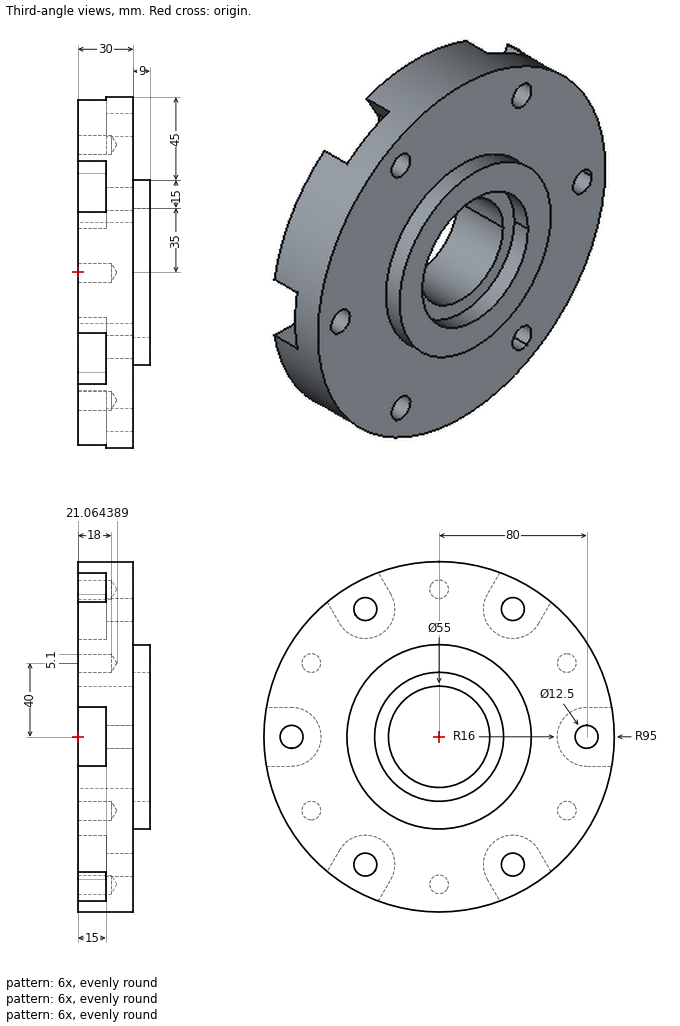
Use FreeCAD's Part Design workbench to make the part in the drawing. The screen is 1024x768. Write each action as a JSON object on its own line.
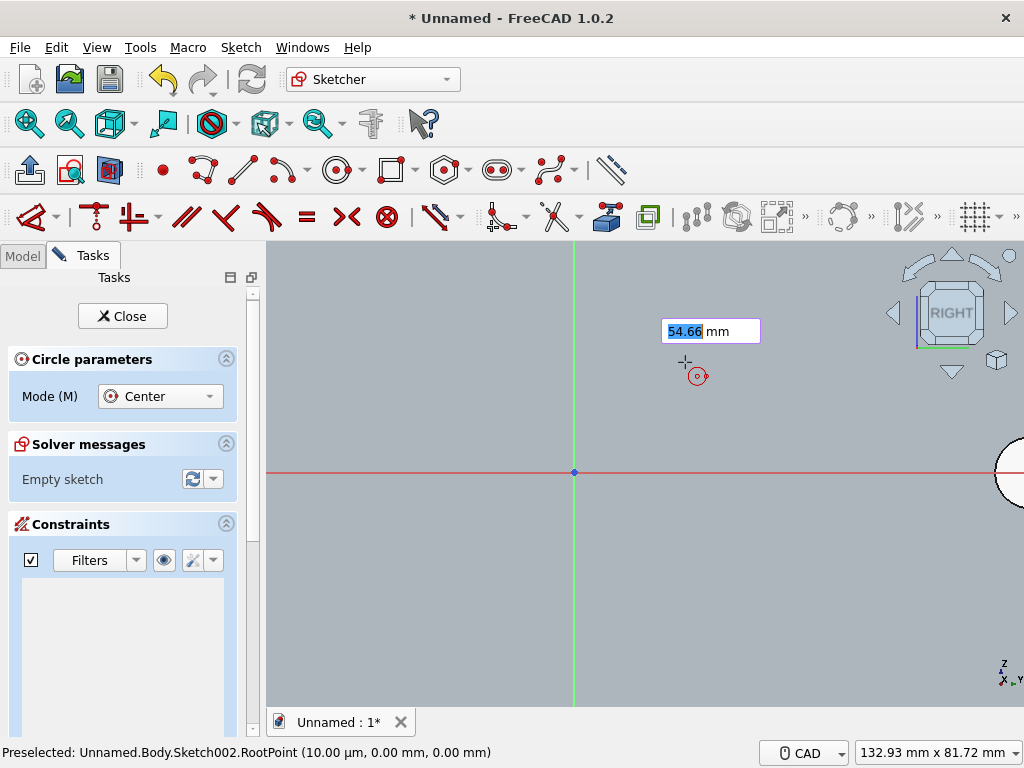
{"action": "type", "text": "55"}
{"action": "key", "text": "Return"}
{"action": "key", "text": "Escape"}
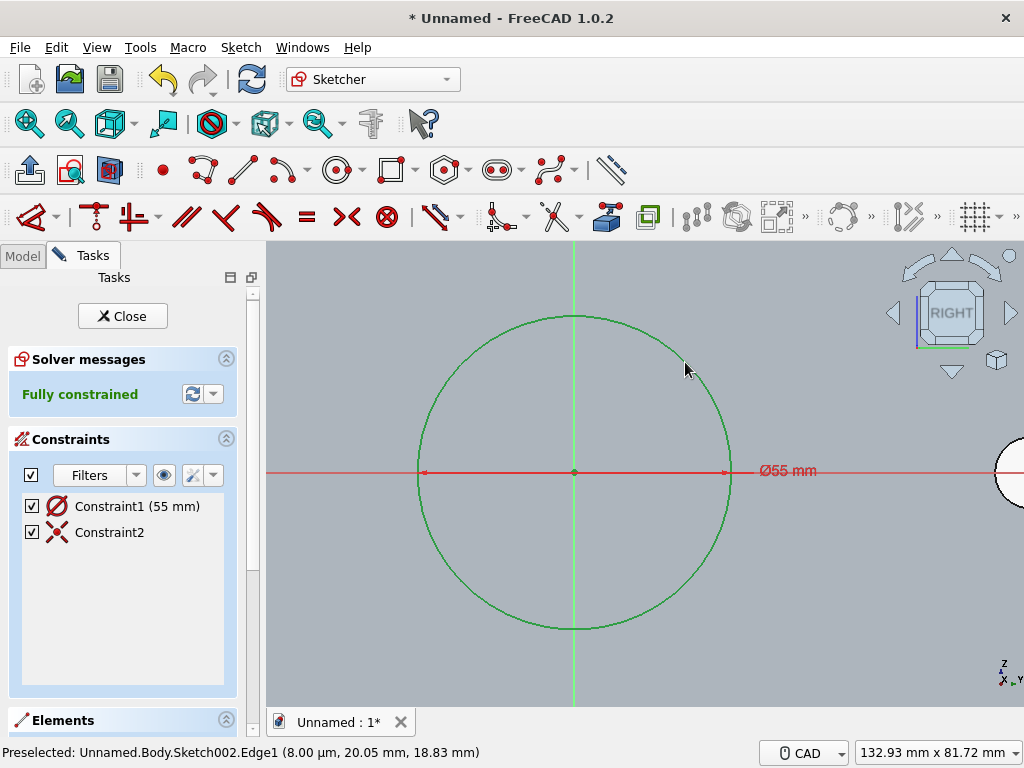
{"action": "left_click", "coordinate": [123, 316]}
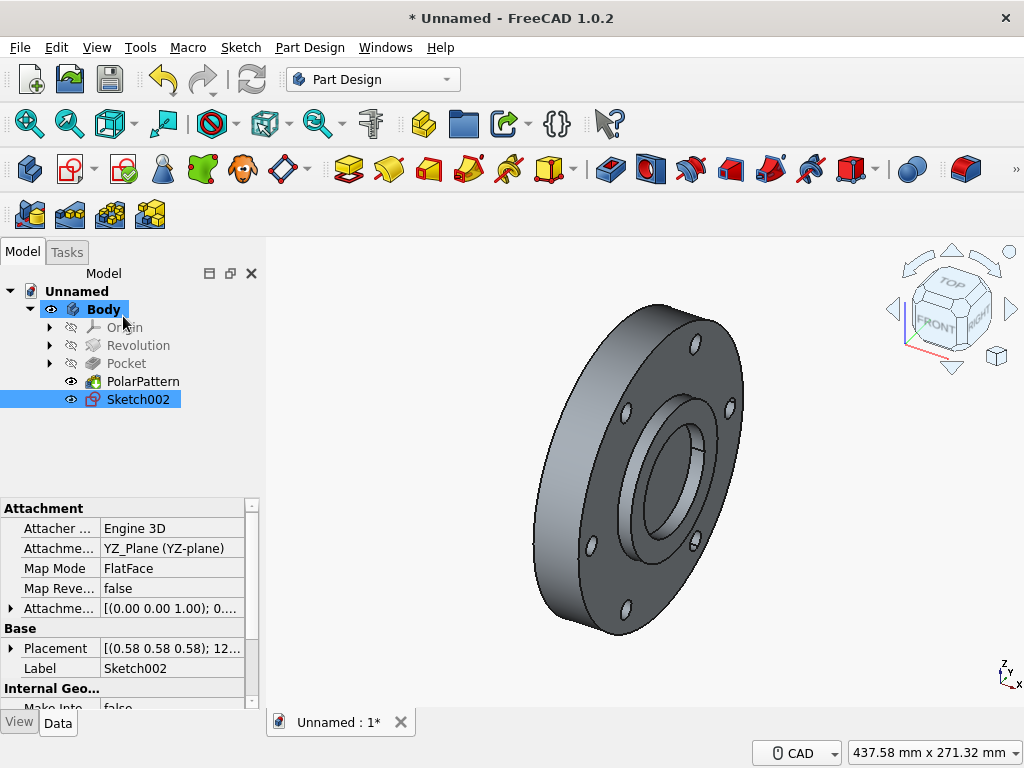
{"action": "left_click", "coordinate": [612, 170]}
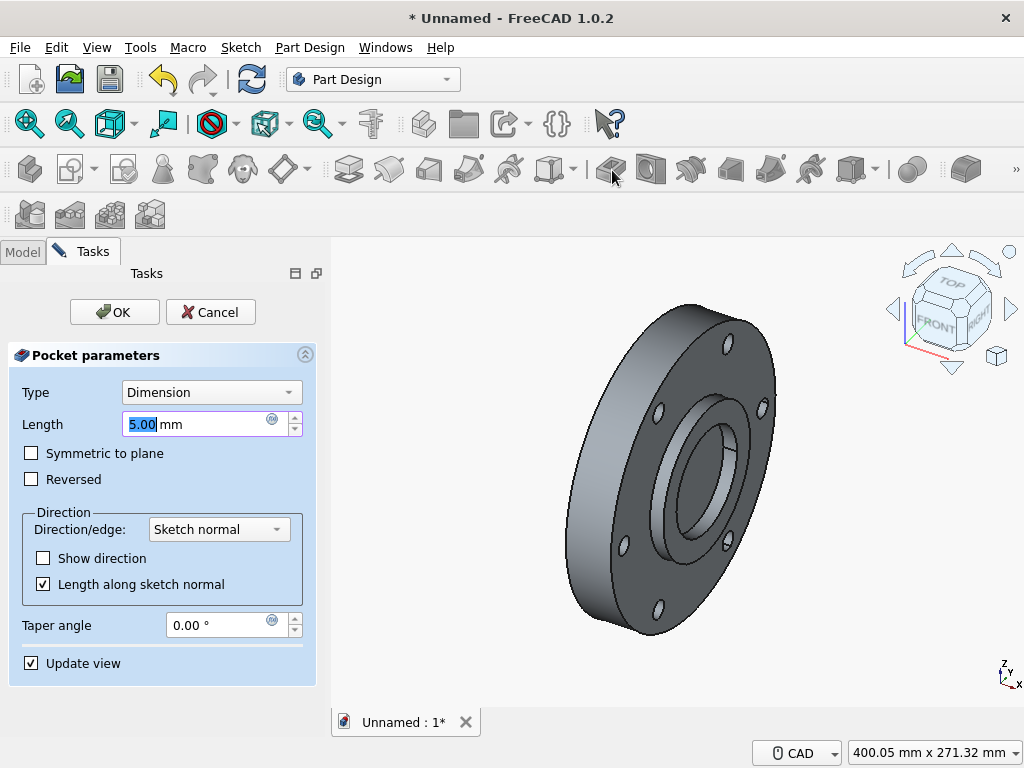
{"action": "left_click", "coordinate": [212, 392]}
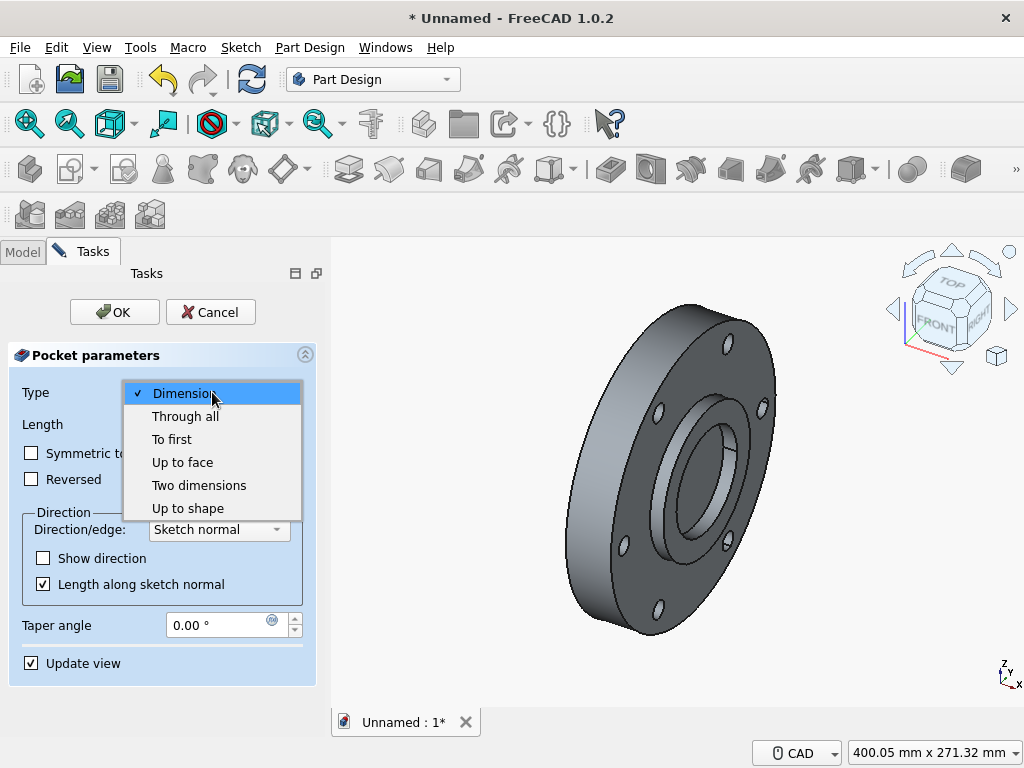
{"action": "left_click", "coordinate": [212, 416]}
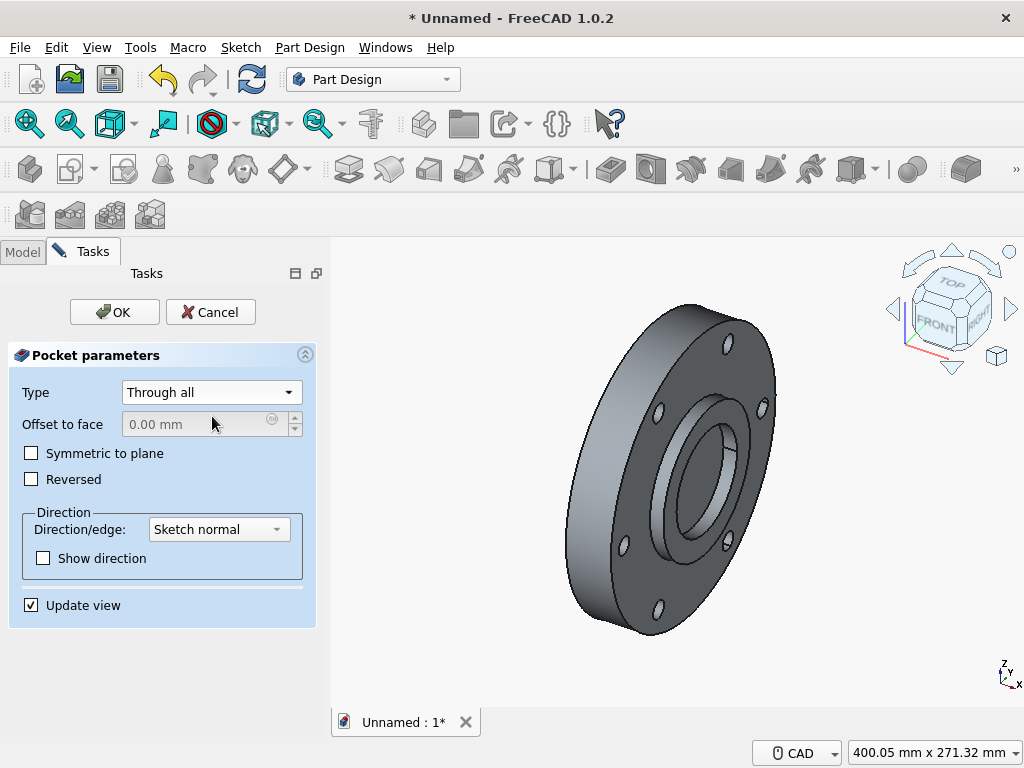
{"action": "left_click", "coordinate": [30, 479]}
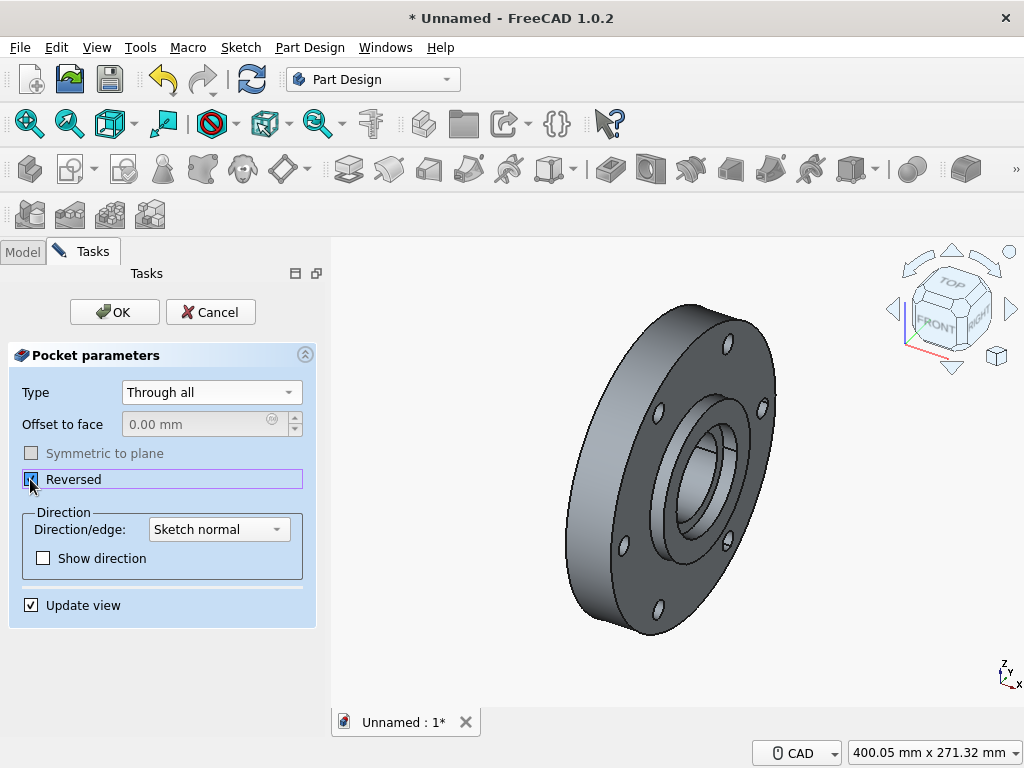
{"action": "left_click", "coordinate": [115, 312]}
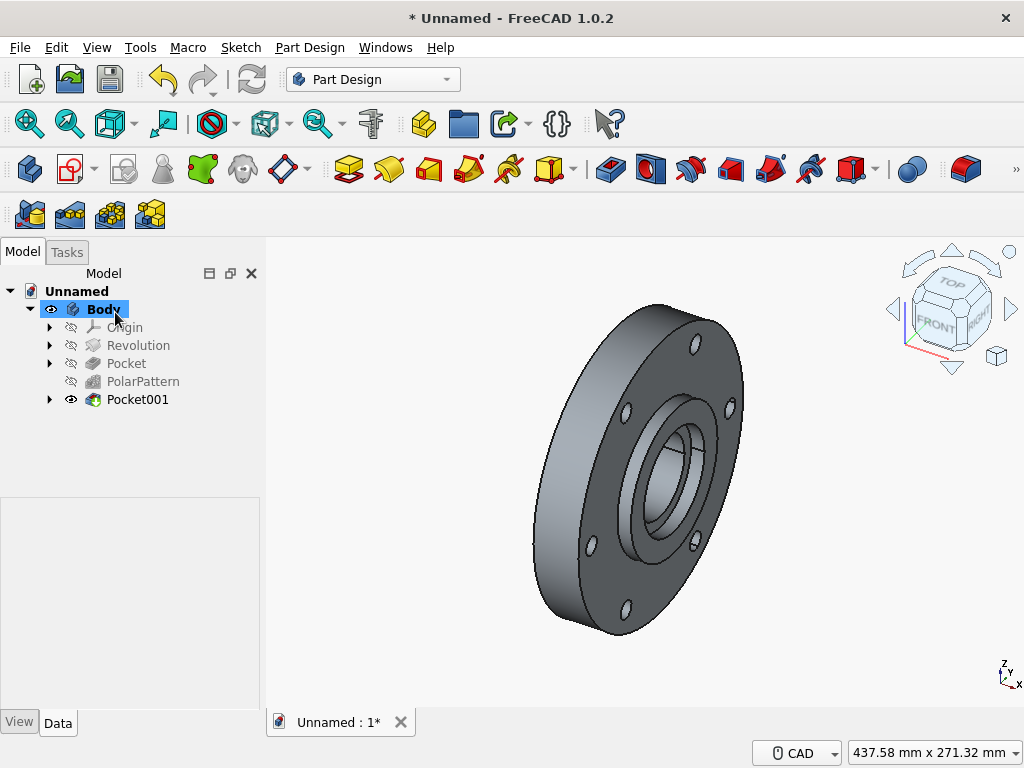
{"action": "left_click", "coordinate": [50, 327]}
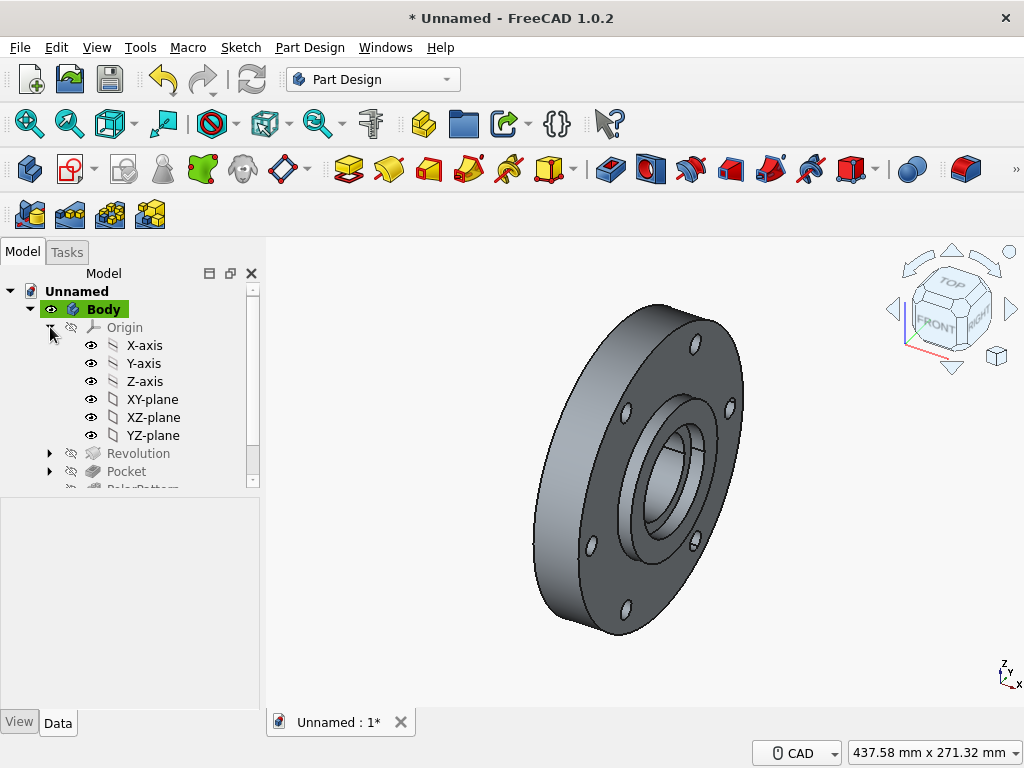
{"action": "left_click", "coordinate": [136, 435]}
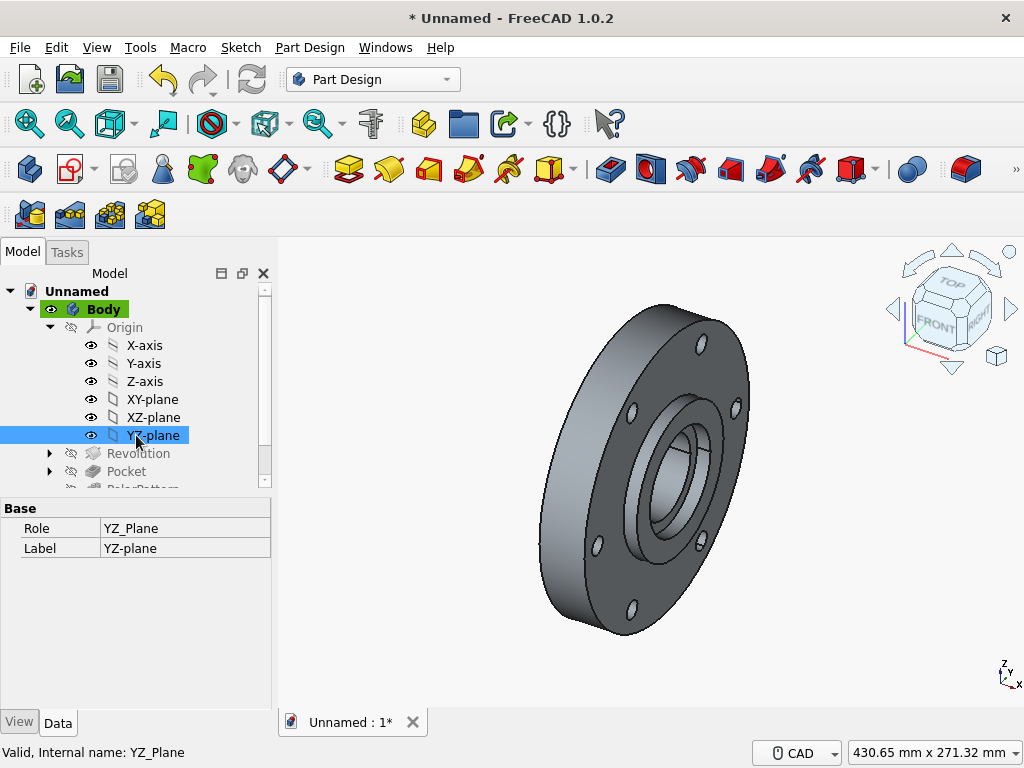
{"action": "left_click", "coordinate": [284, 170]}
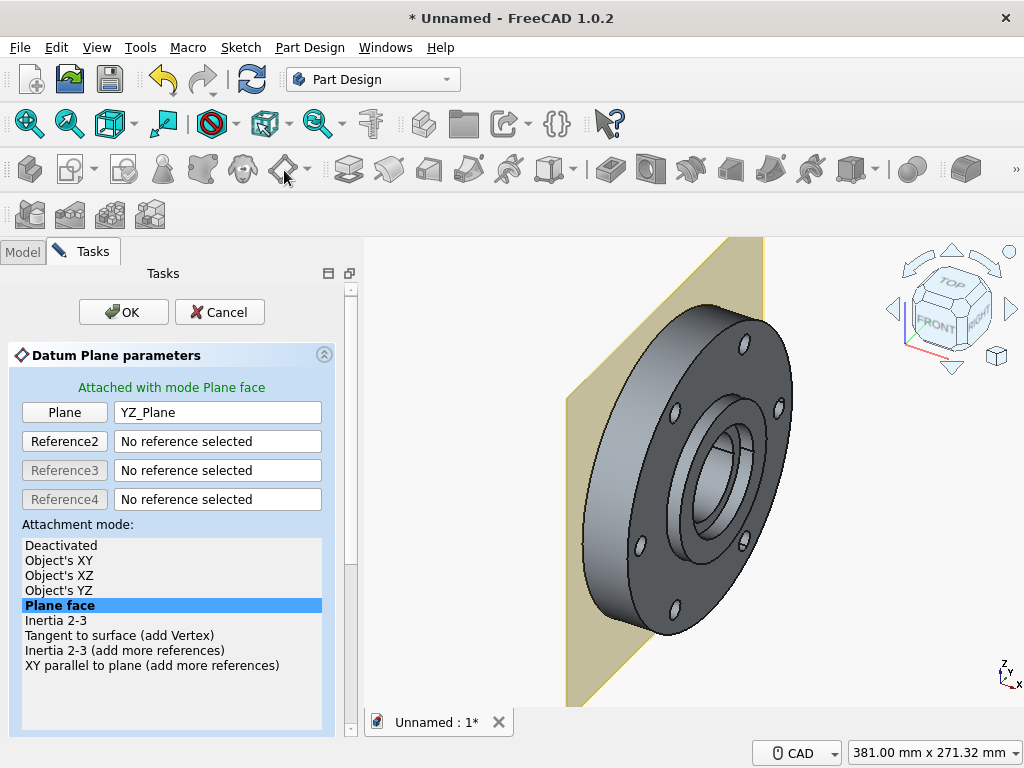
{"action": "scroll", "coordinate": [351, 510], "scroll_direction": "down", "scroll_amount": 3}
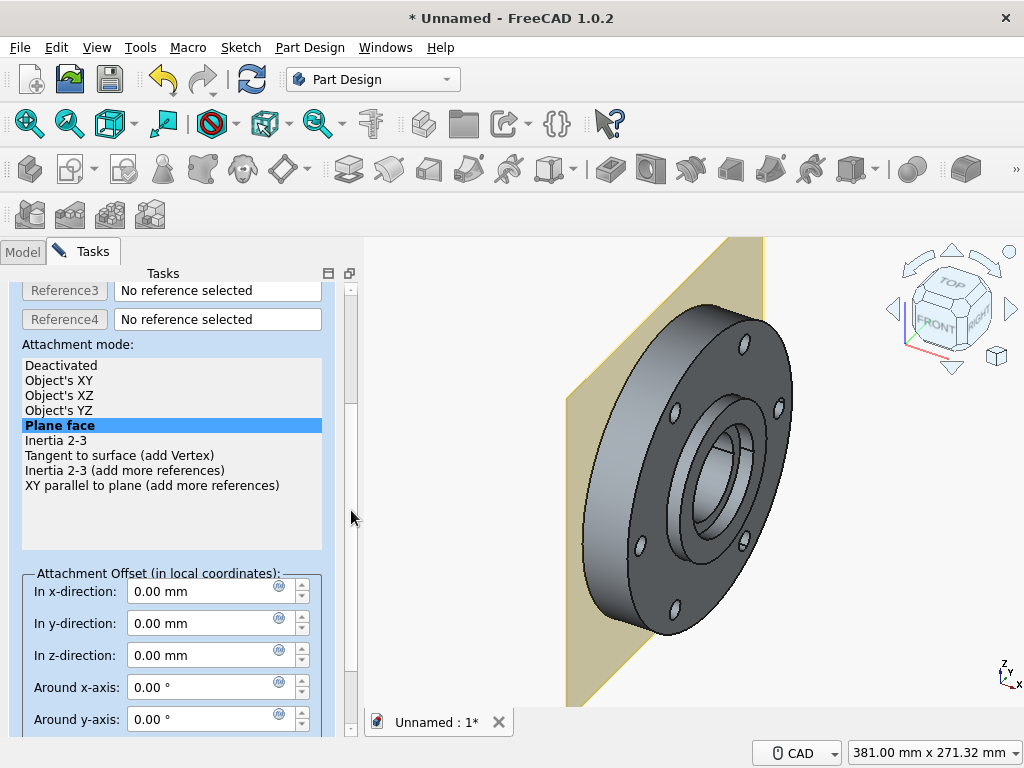
{"action": "triple_click", "coordinate": [210, 655]}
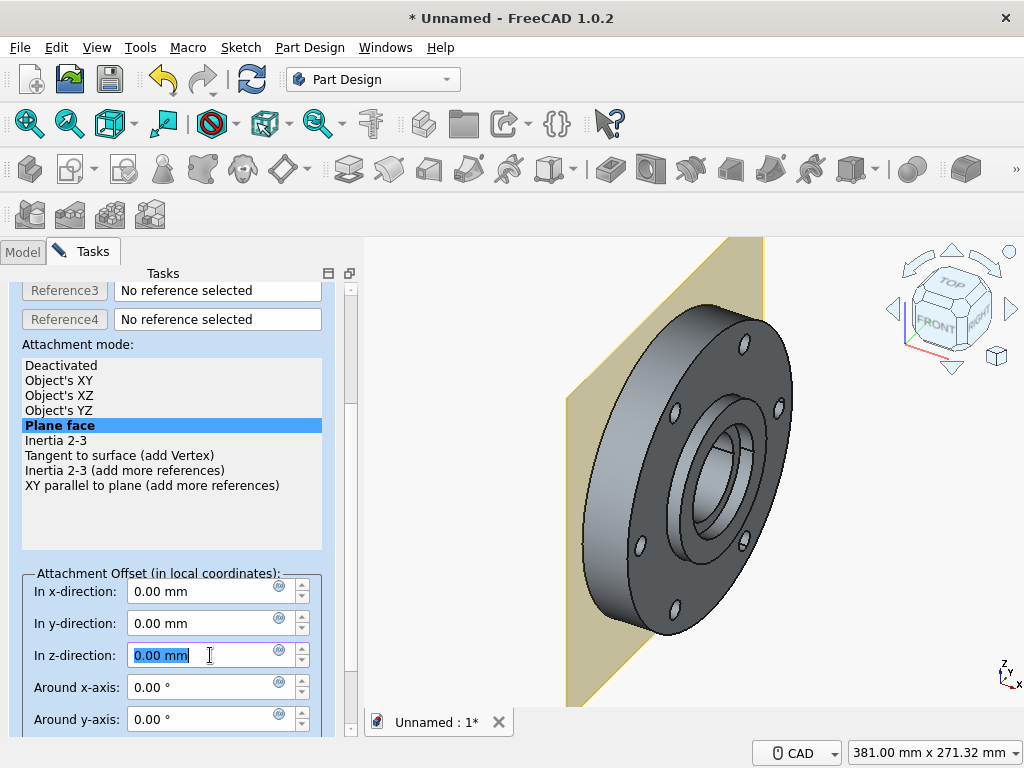
{"action": "type", "text": "15"}
{"action": "key", "text": "Tab"}